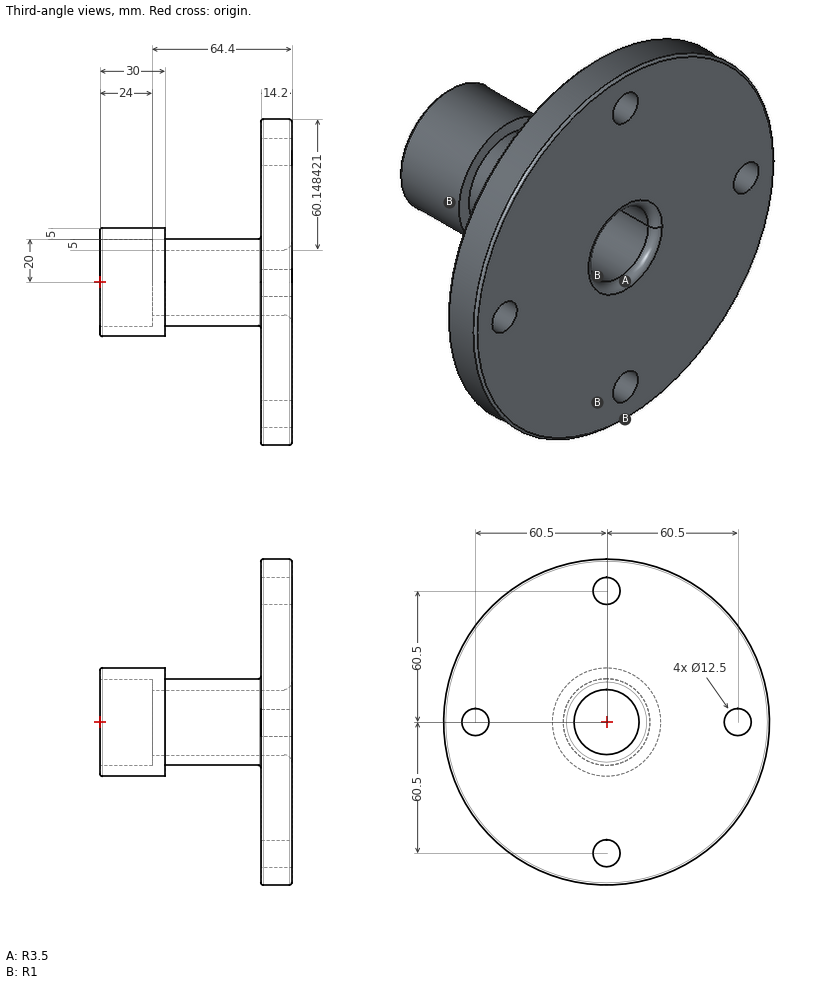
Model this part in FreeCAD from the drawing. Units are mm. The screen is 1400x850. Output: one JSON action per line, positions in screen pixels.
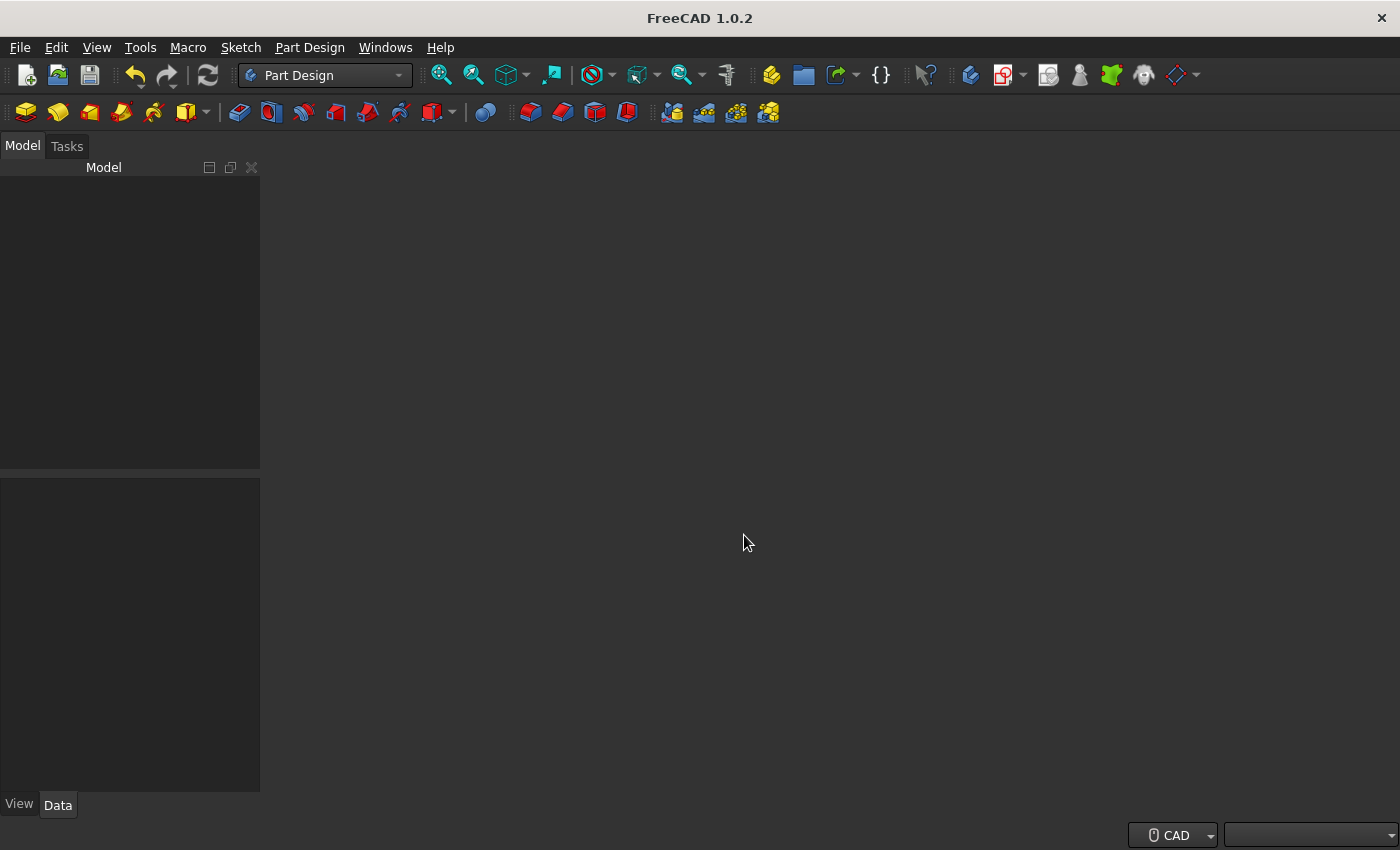
{"action": "key", "text": "ctrl+n"}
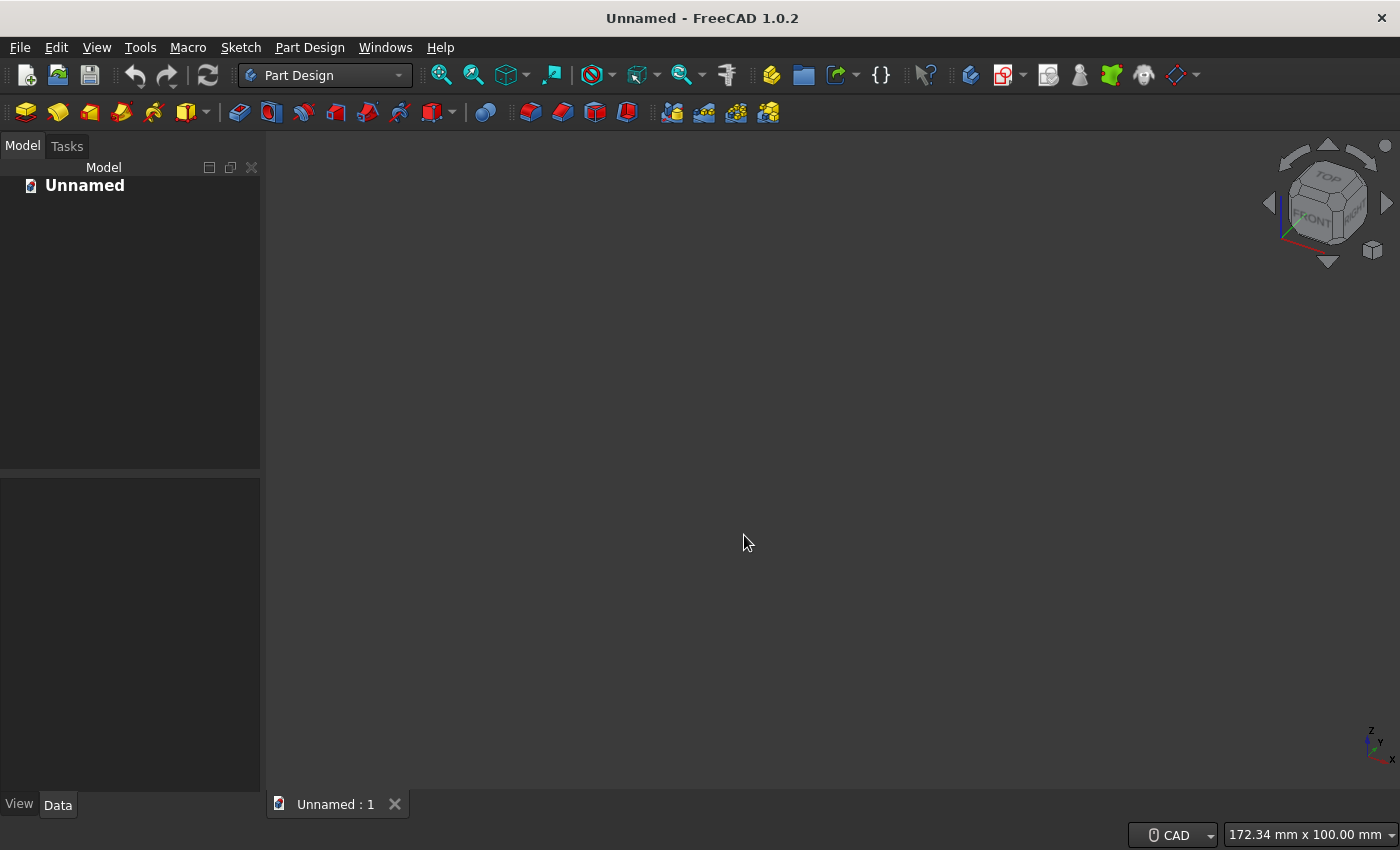
{"action": "left_click", "coordinate": [1004, 76]}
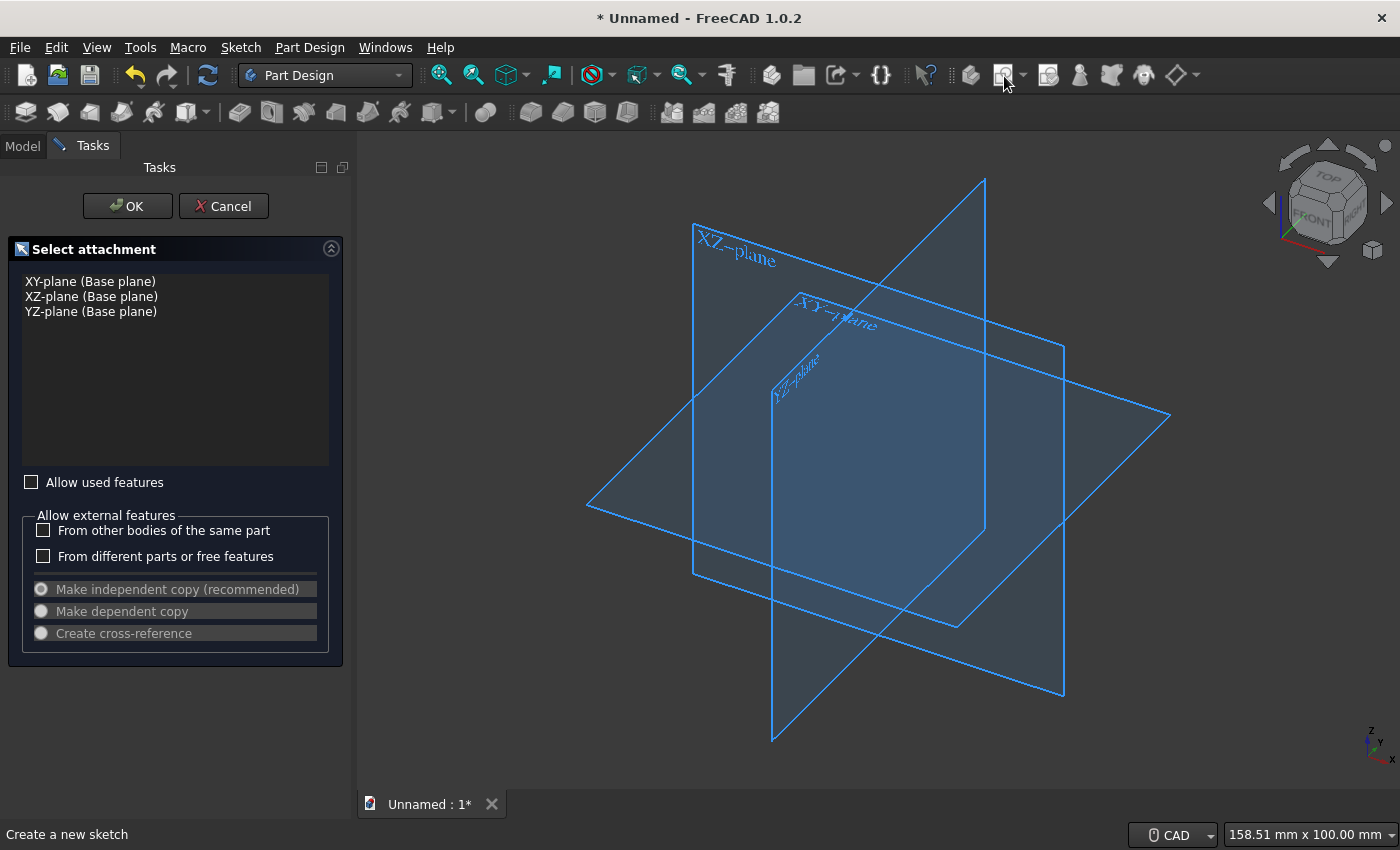
{"action": "left_click", "coordinate": [82, 282]}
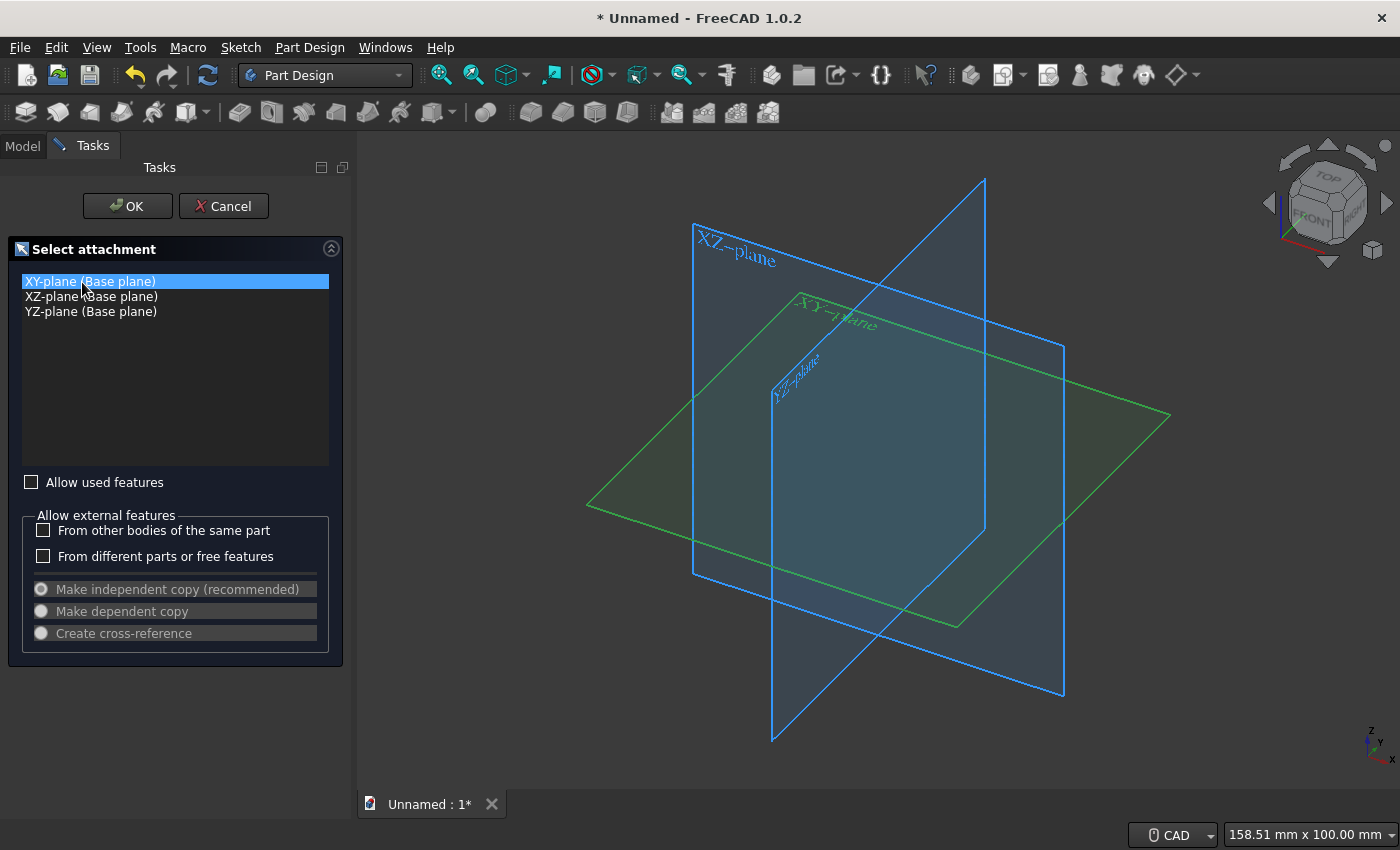
{"action": "left_click", "coordinate": [128, 206]}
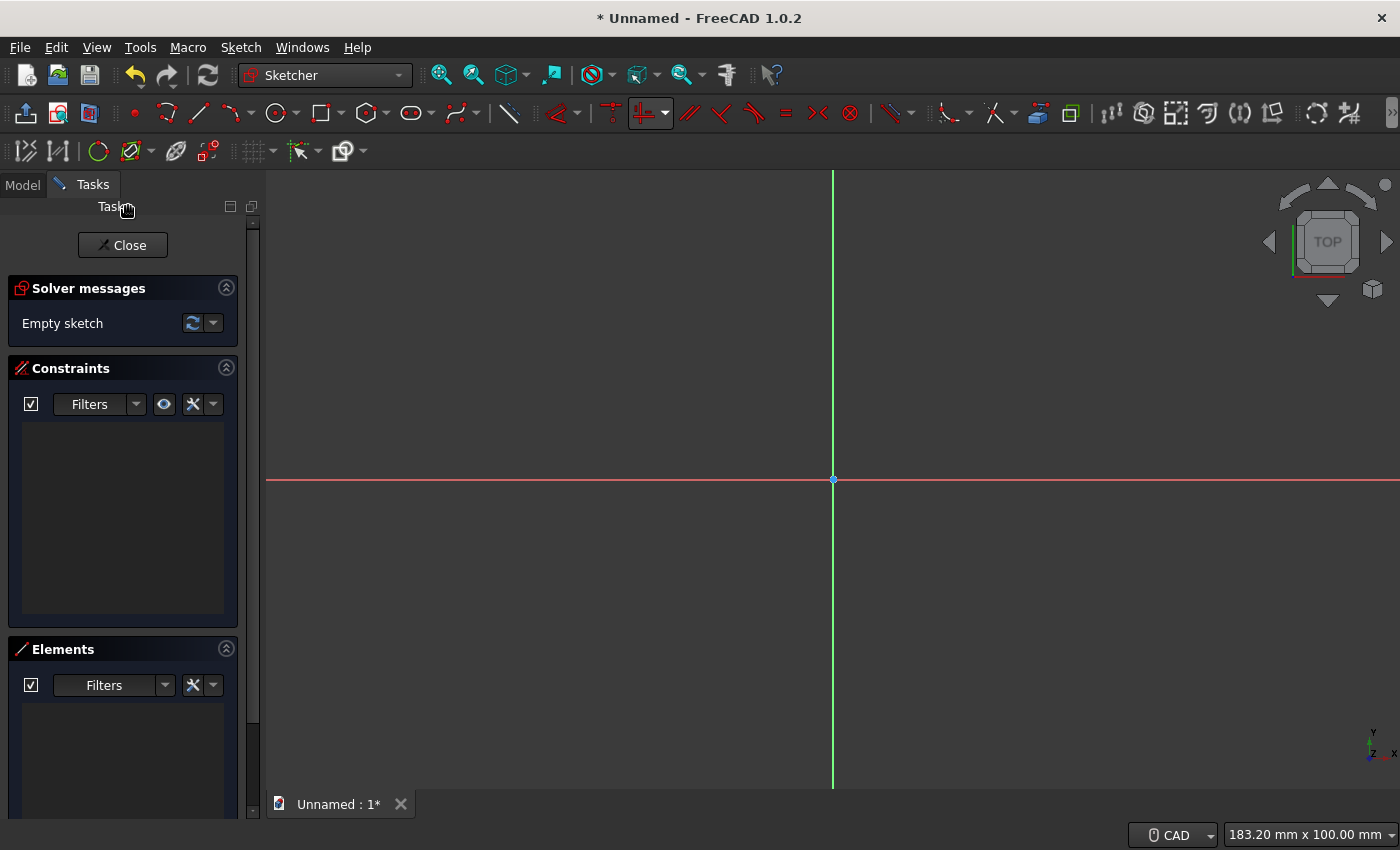
{"action": "scroll", "coordinate": [294, 761], "scroll_direction": "down", "scroll_amount": 2}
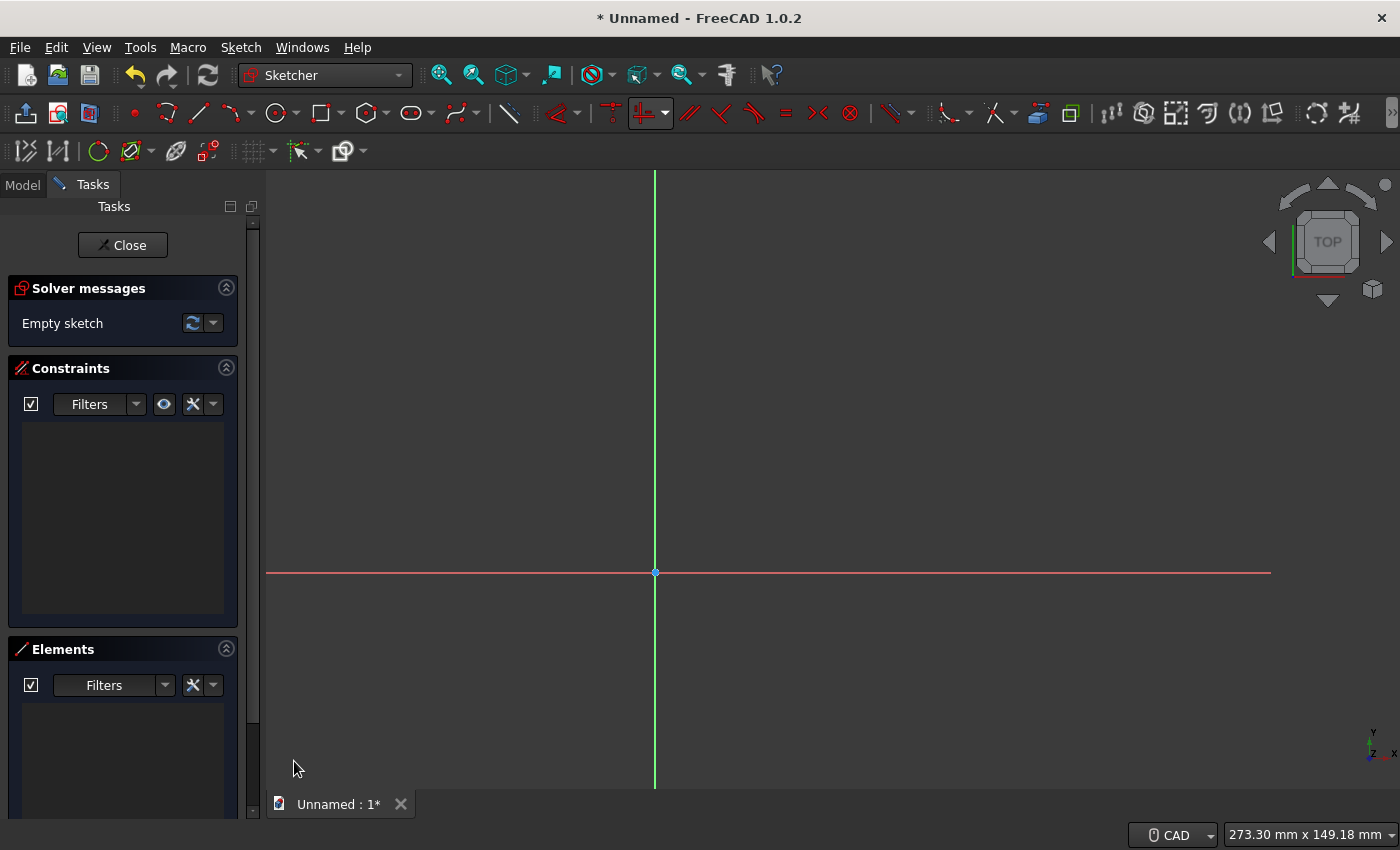
{"action": "key", "text": "g m"}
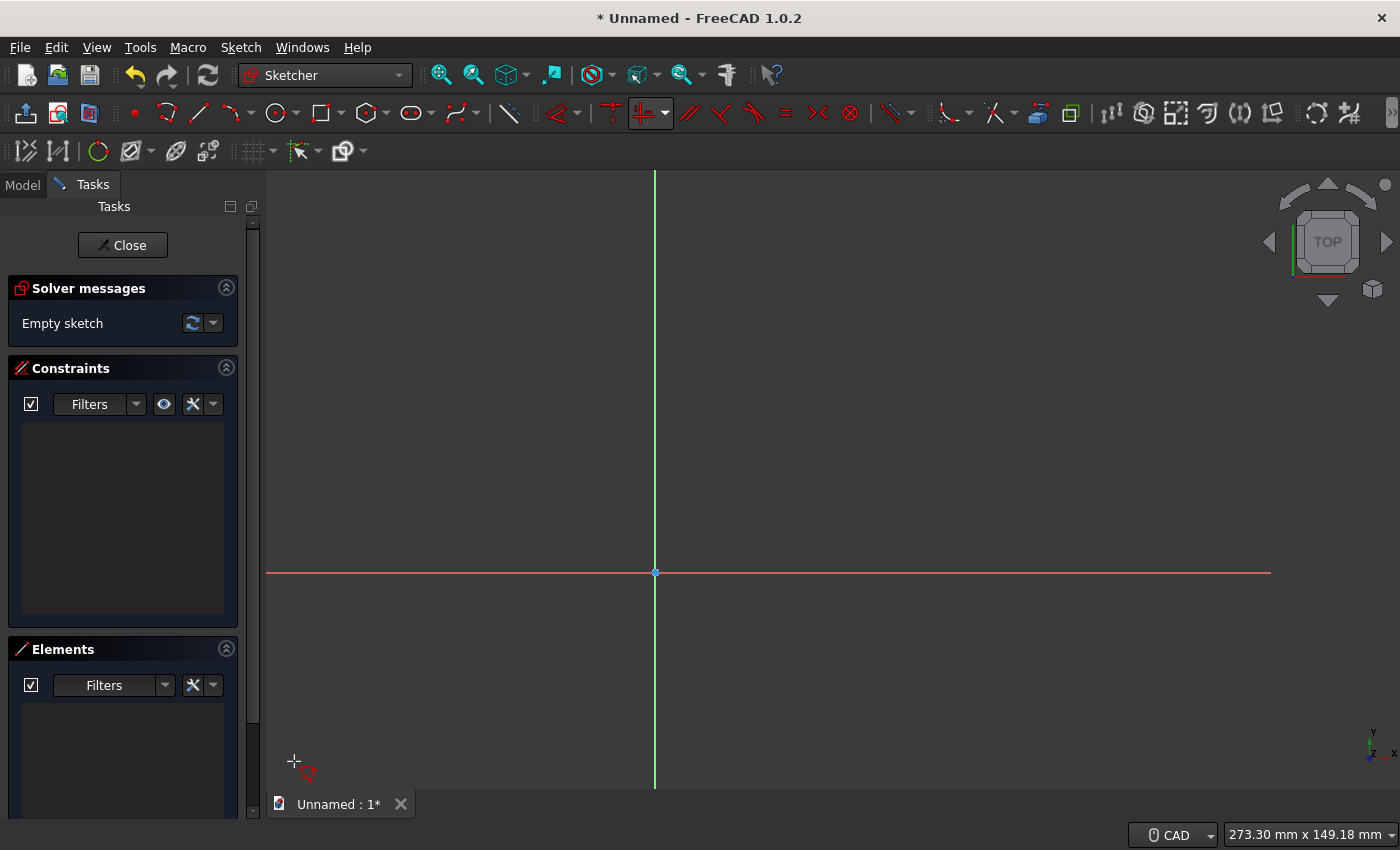
{"action": "left_click", "coordinate": [655, 490]}
{"action": "left_click", "coordinate": [755, 490]}
{"action": "left_click", "coordinate": [755, 510]}
{"action": "left_click", "coordinate": [1022, 510]}
{"action": "left_click", "coordinate": [1022, 261]}
{"action": "left_click", "coordinate": [963, 261]}
{"action": "left_click", "coordinate": [963, 490]}
{"action": "left_click", "coordinate": [780, 490]}
{"action": "left_click", "coordinate": [780, 469]}
{"action": "left_click", "coordinate": [664, 469]}
{"action": "left_click", "coordinate": [655, 491]}
{"action": "key", "text": "Escape"}
{"action": "key", "text": "Escape"}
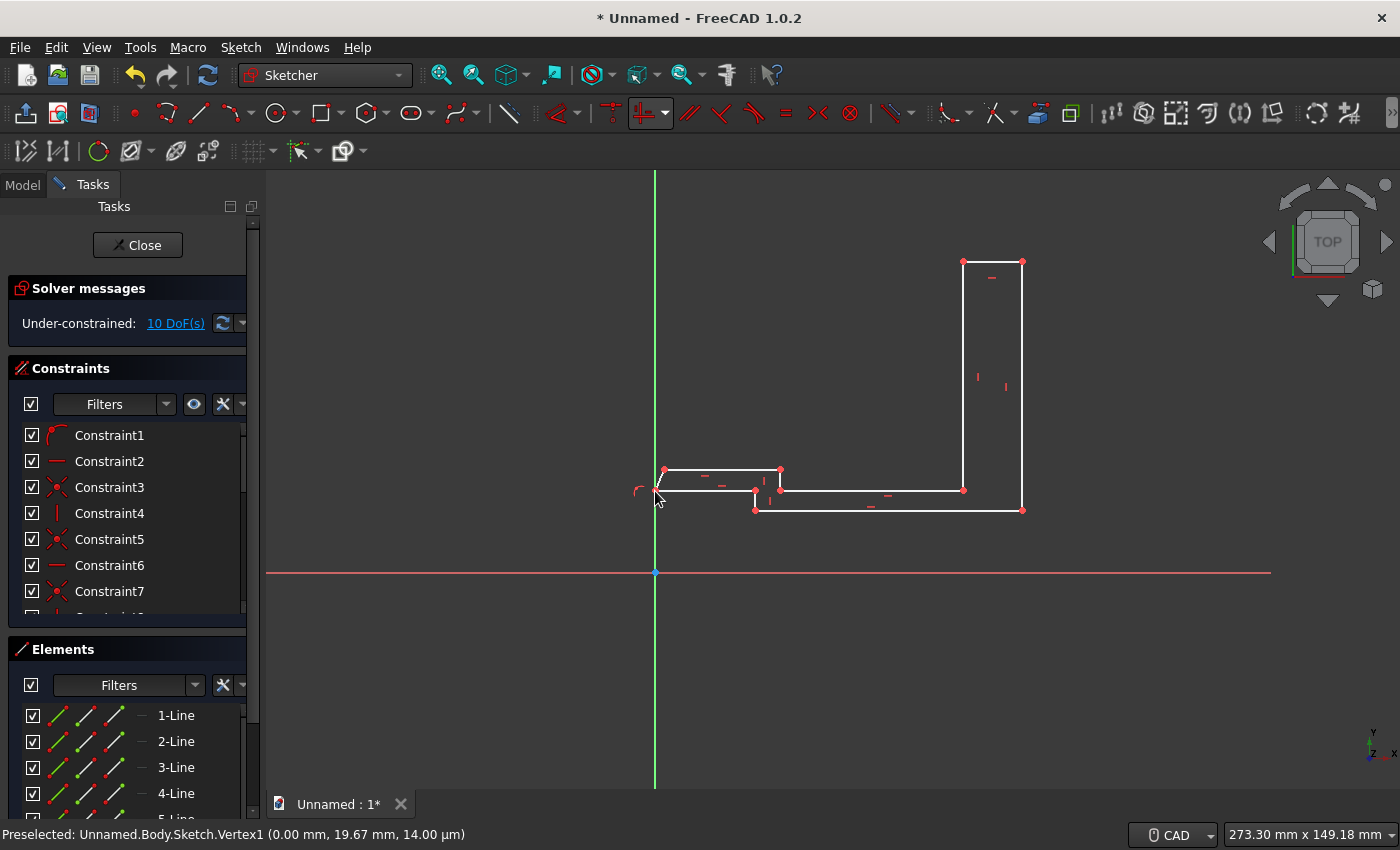
{"action": "scroll", "coordinate": [659, 483], "scroll_direction": "up", "scroll_amount": 3}